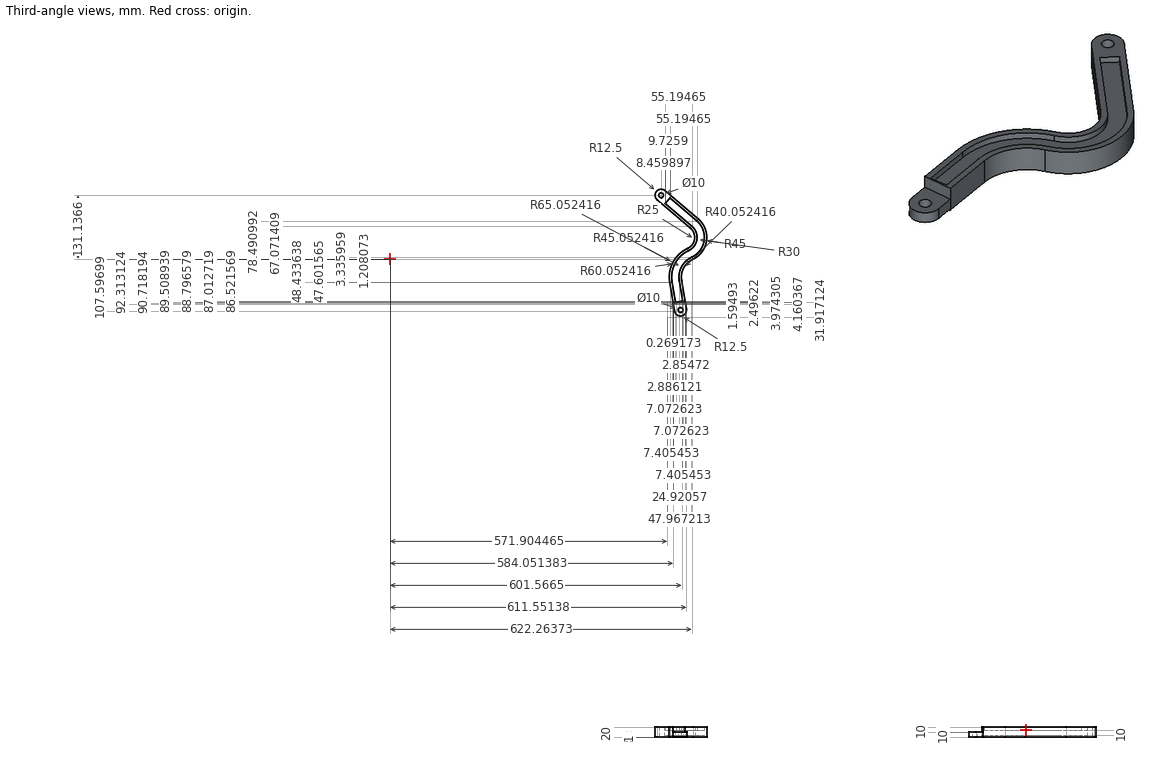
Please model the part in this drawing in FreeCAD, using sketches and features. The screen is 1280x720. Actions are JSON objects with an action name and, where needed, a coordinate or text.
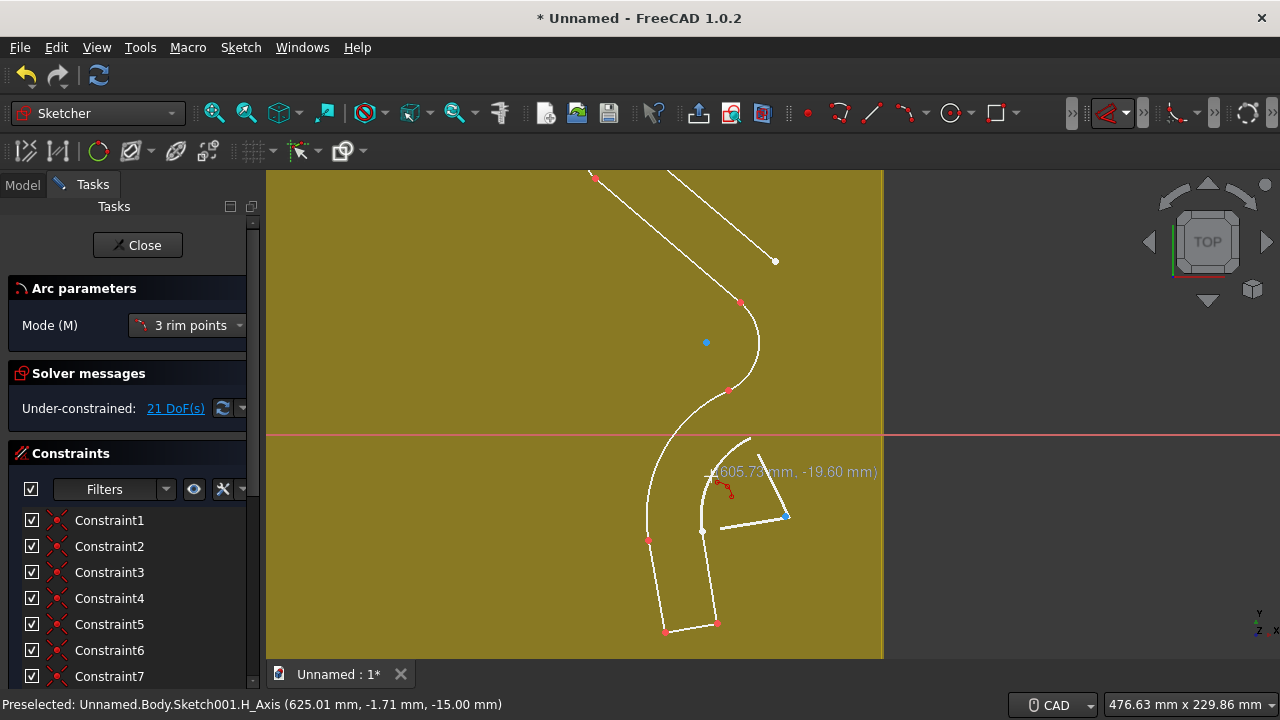
{"action": "left_click", "coordinate": [711, 476]}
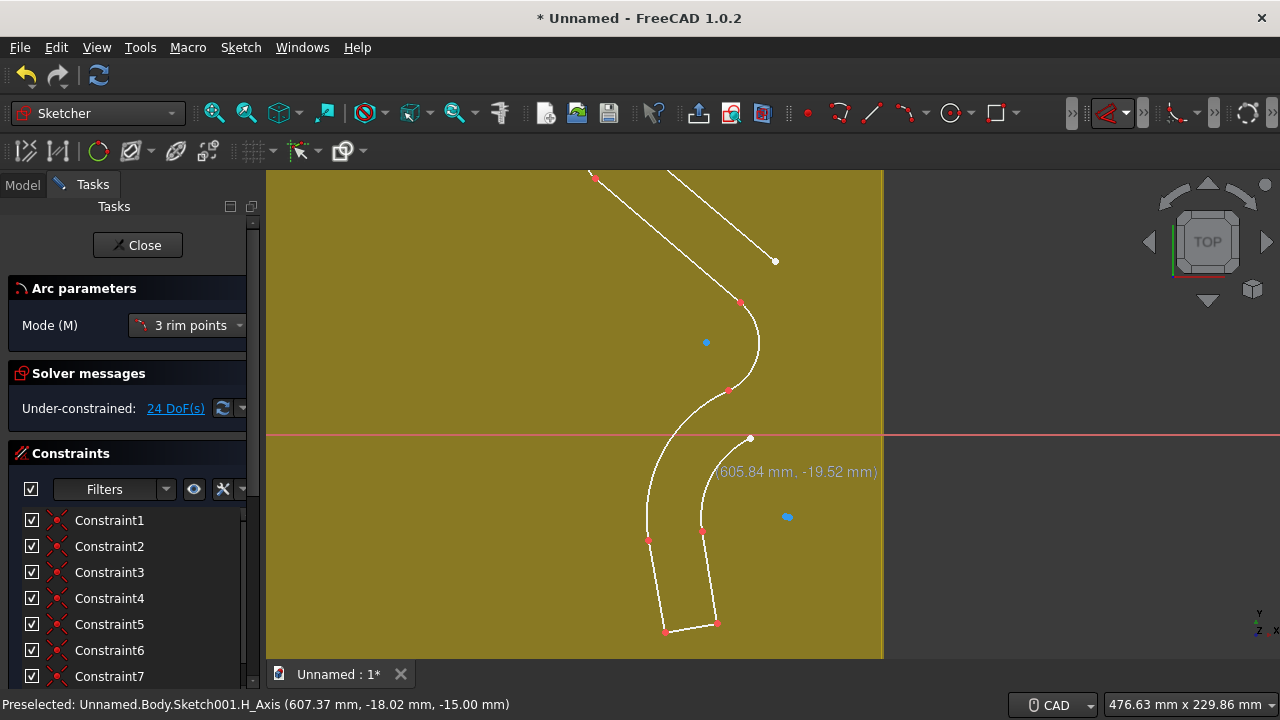
{"action": "scroll", "coordinate": [750, 438], "scroll_direction": "up", "scroll_amount": 10}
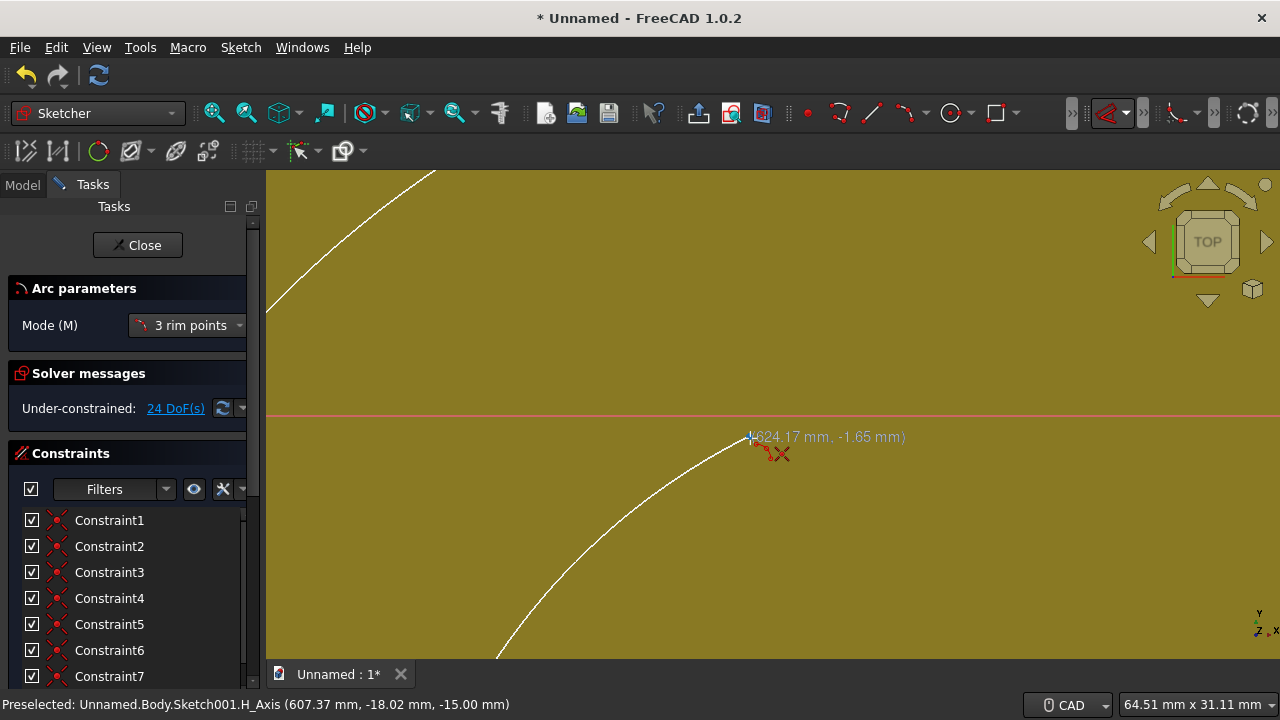
{"action": "left_click", "coordinate": [749, 436]}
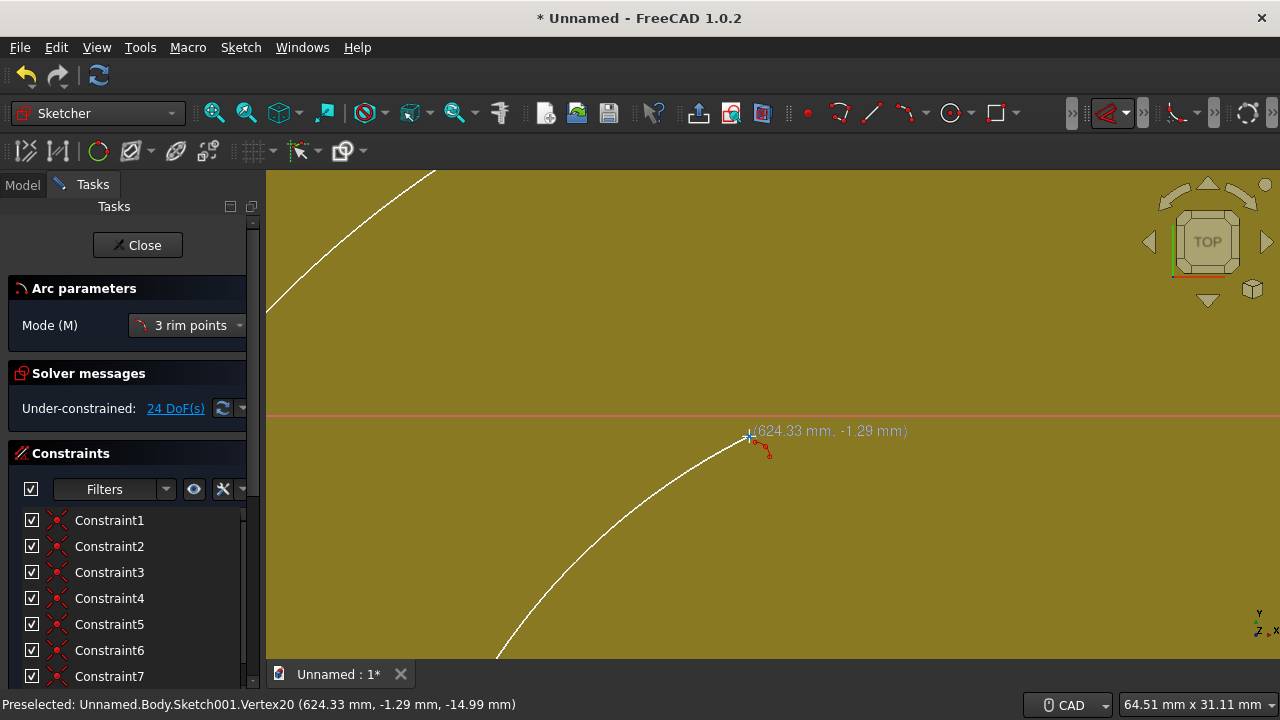
{"action": "scroll", "coordinate": [736, 452], "scroll_direction": "down", "scroll_amount": 12}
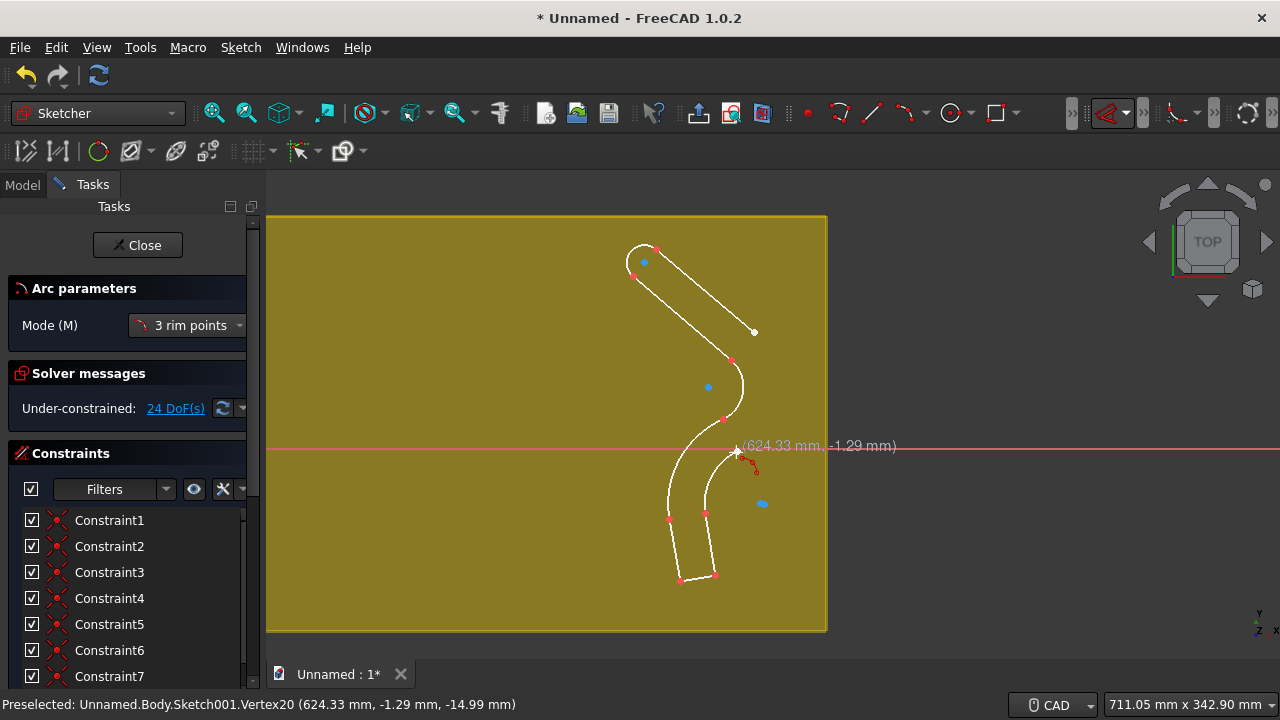
{"action": "left_click", "coordinate": [754, 333]}
{"action": "left_click", "coordinate": [779, 396]}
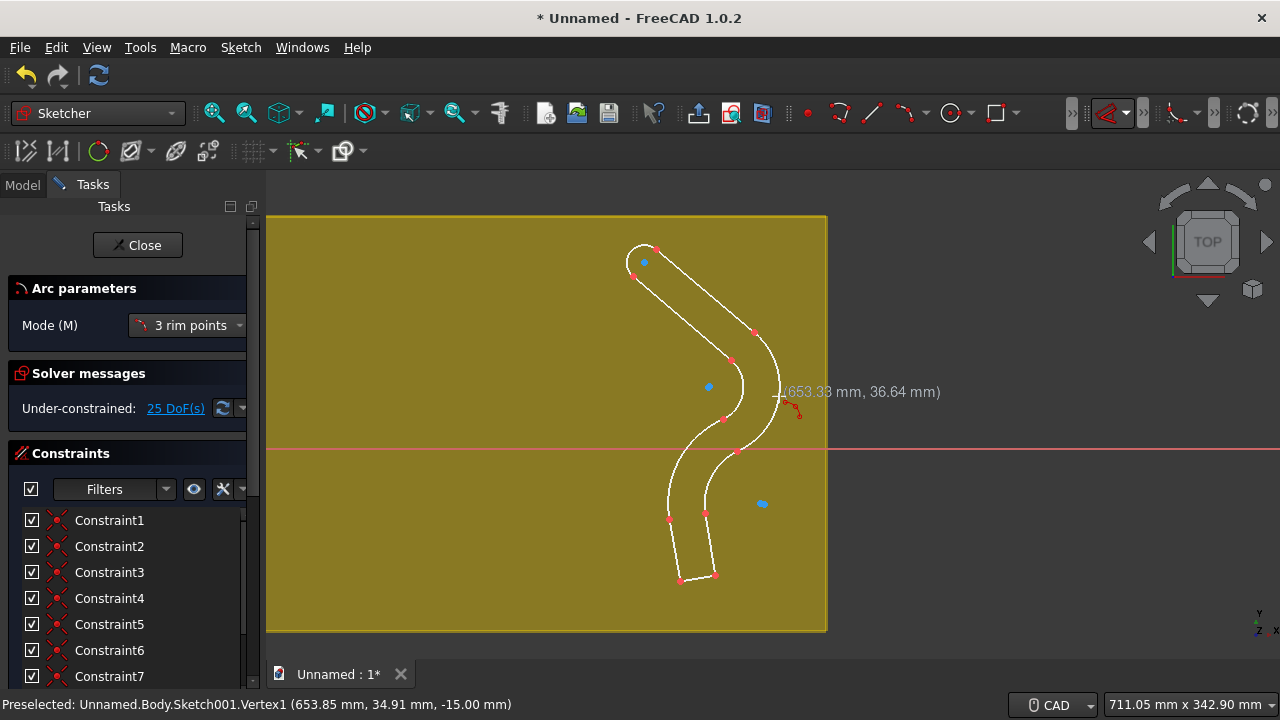
{"action": "key", "text": "g m"}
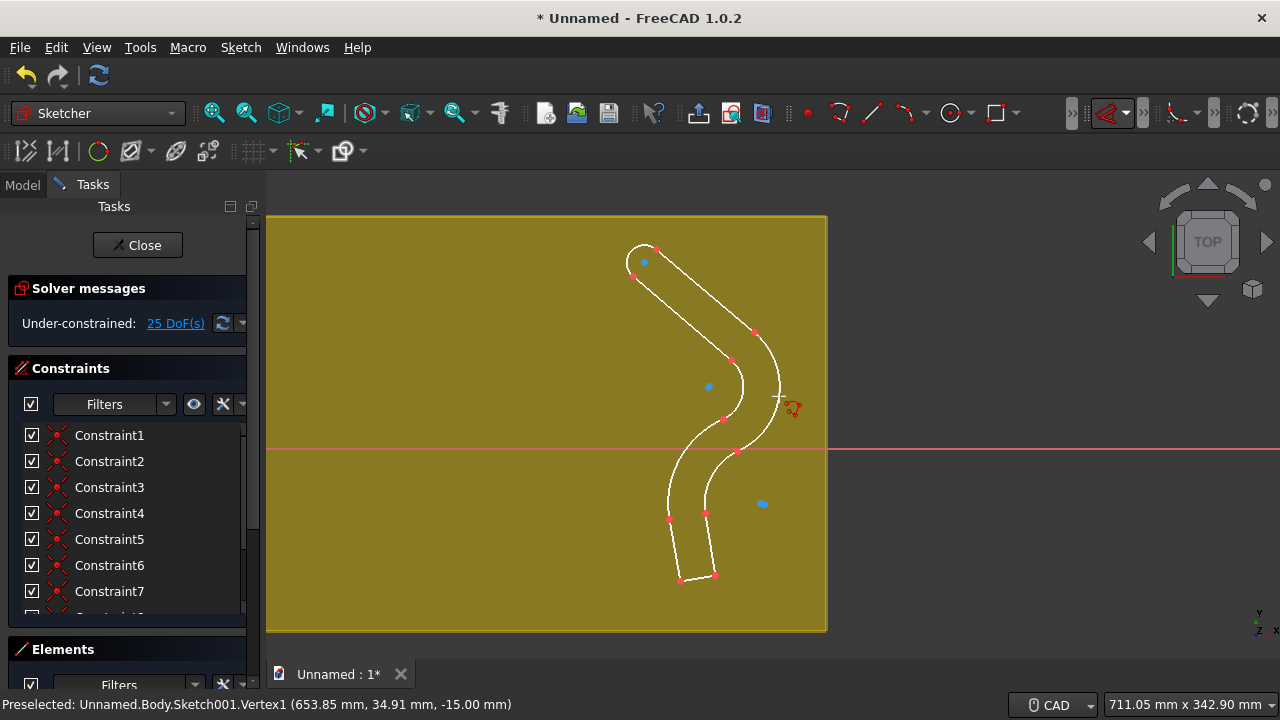
{"action": "scroll", "coordinate": [698, 514], "scroll_direction": "up", "scroll_amount": 5}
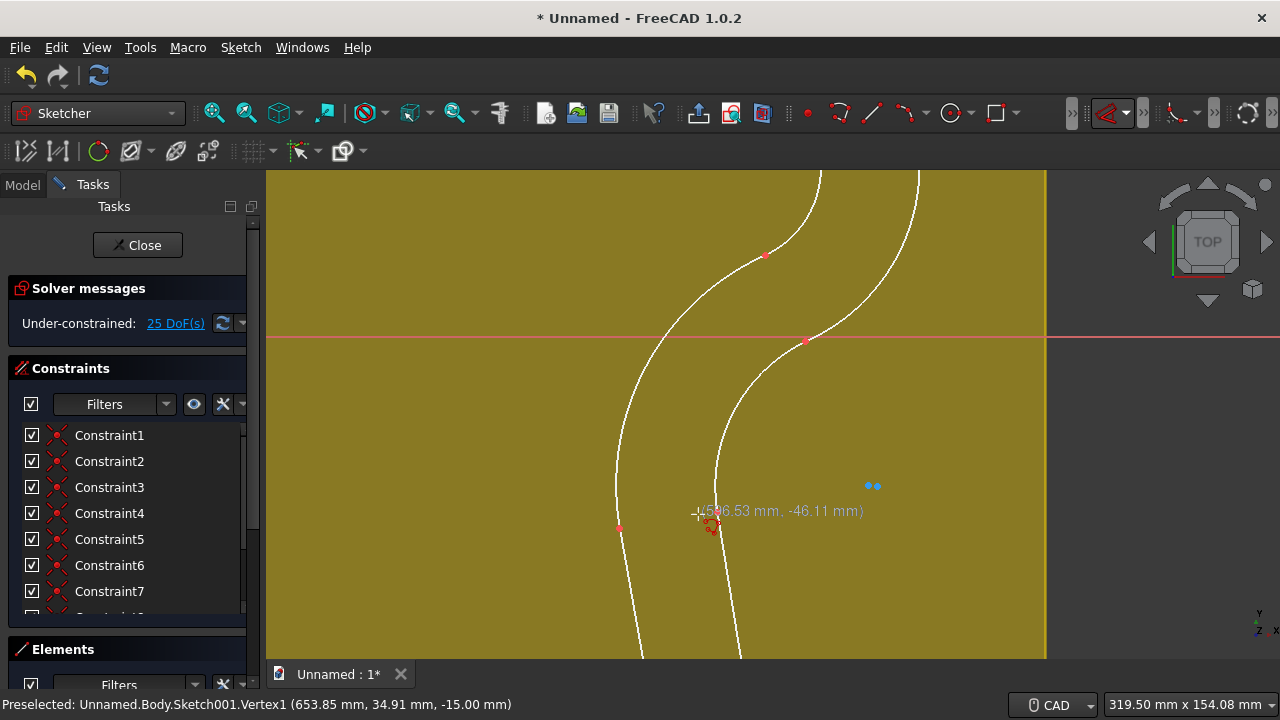
{"action": "left_click", "coordinate": [698, 512]}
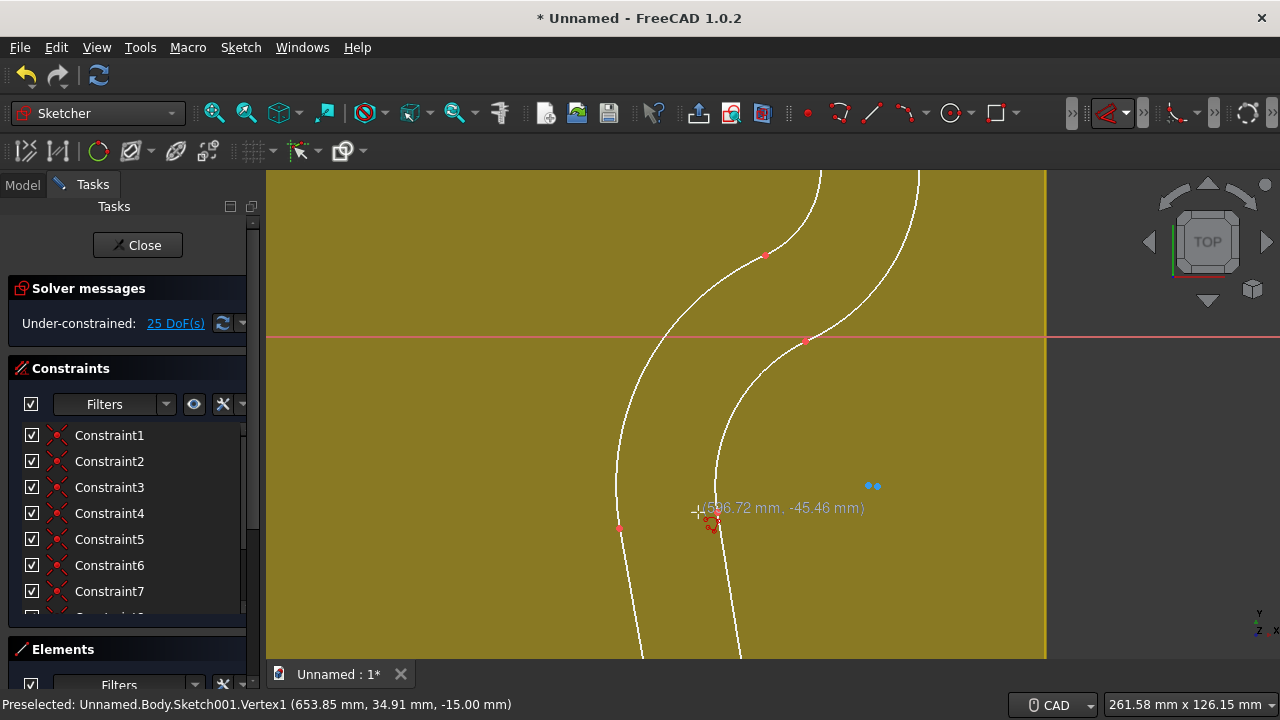
{"action": "scroll", "coordinate": [698, 514], "scroll_direction": "down", "scroll_amount": 5}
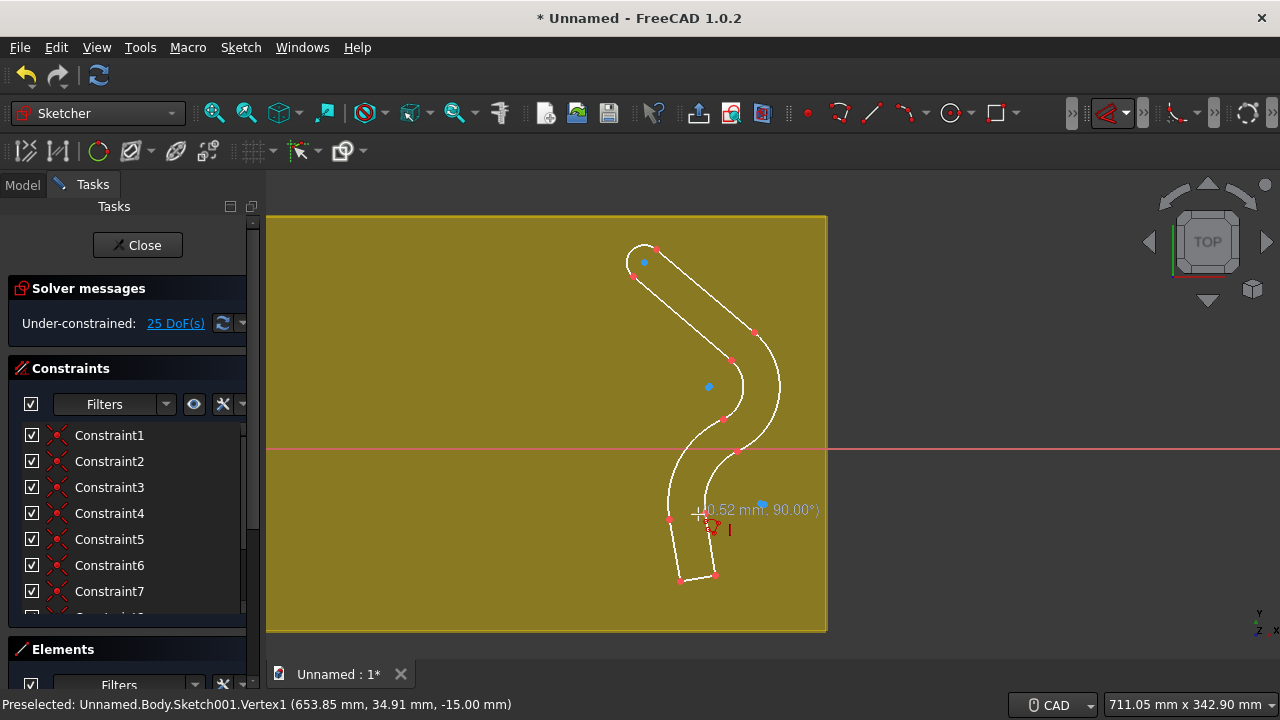
{"action": "scroll", "coordinate": [708, 573], "scroll_direction": "up", "scroll_amount": 9}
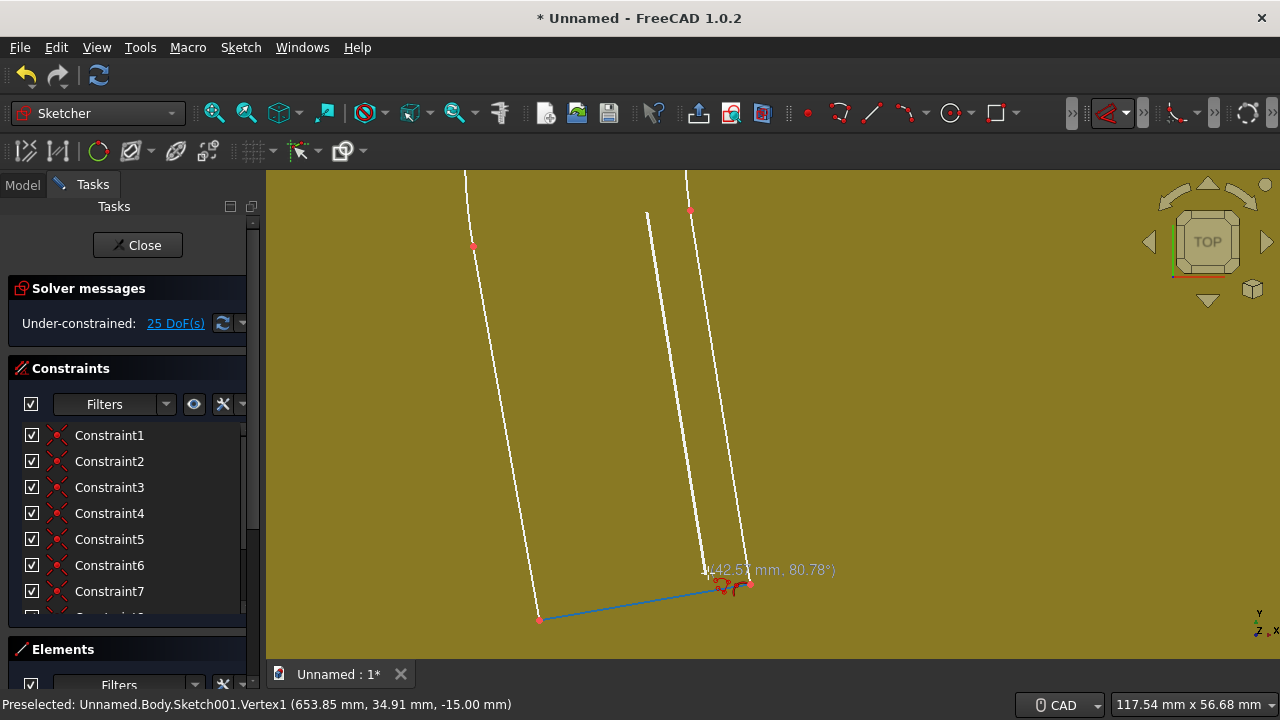
{"action": "left_click", "coordinate": [707, 571]}
{"action": "left_click", "coordinate": [580, 592]}
{"action": "left_click", "coordinate": [519, 231]}
{"action": "right_click", "coordinate": [519, 231]}